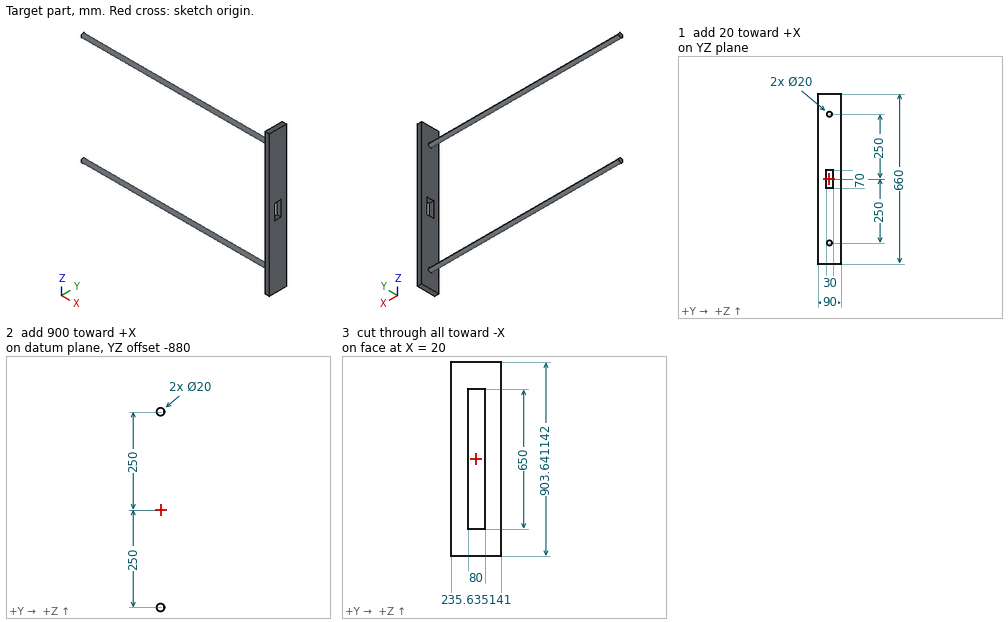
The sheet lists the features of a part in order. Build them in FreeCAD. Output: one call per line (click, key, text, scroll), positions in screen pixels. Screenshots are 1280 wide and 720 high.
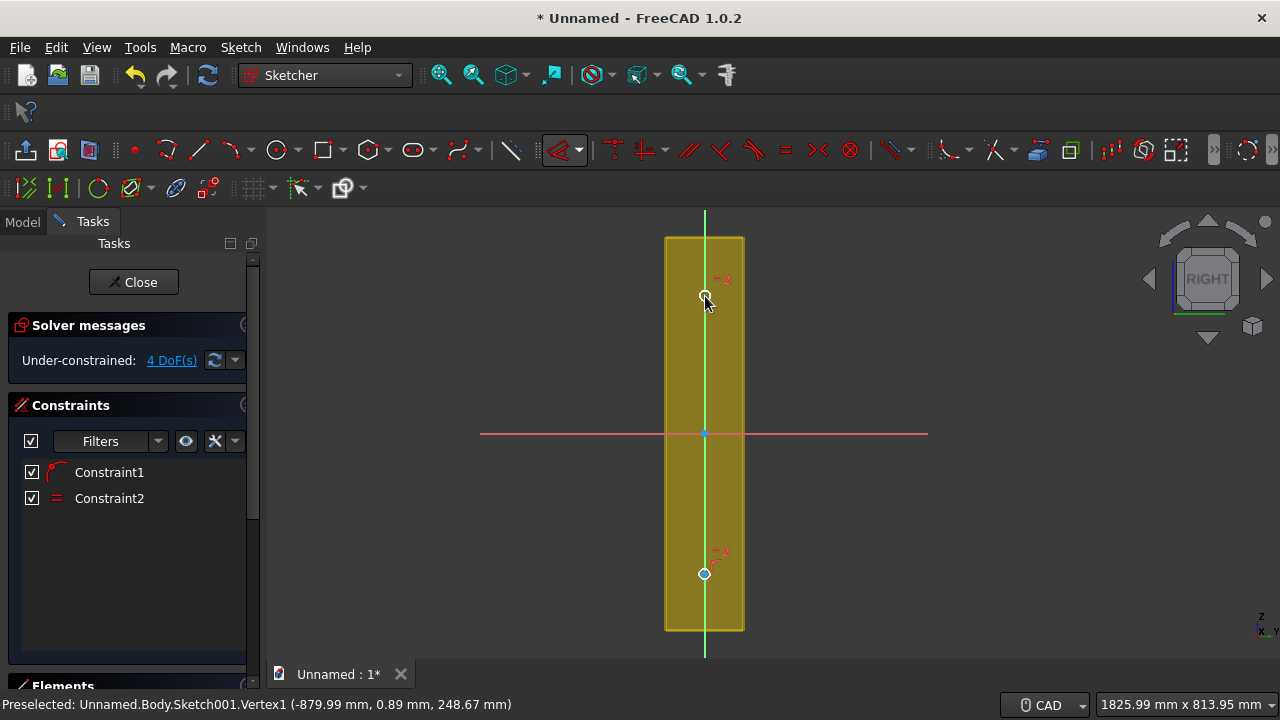
click(705, 518)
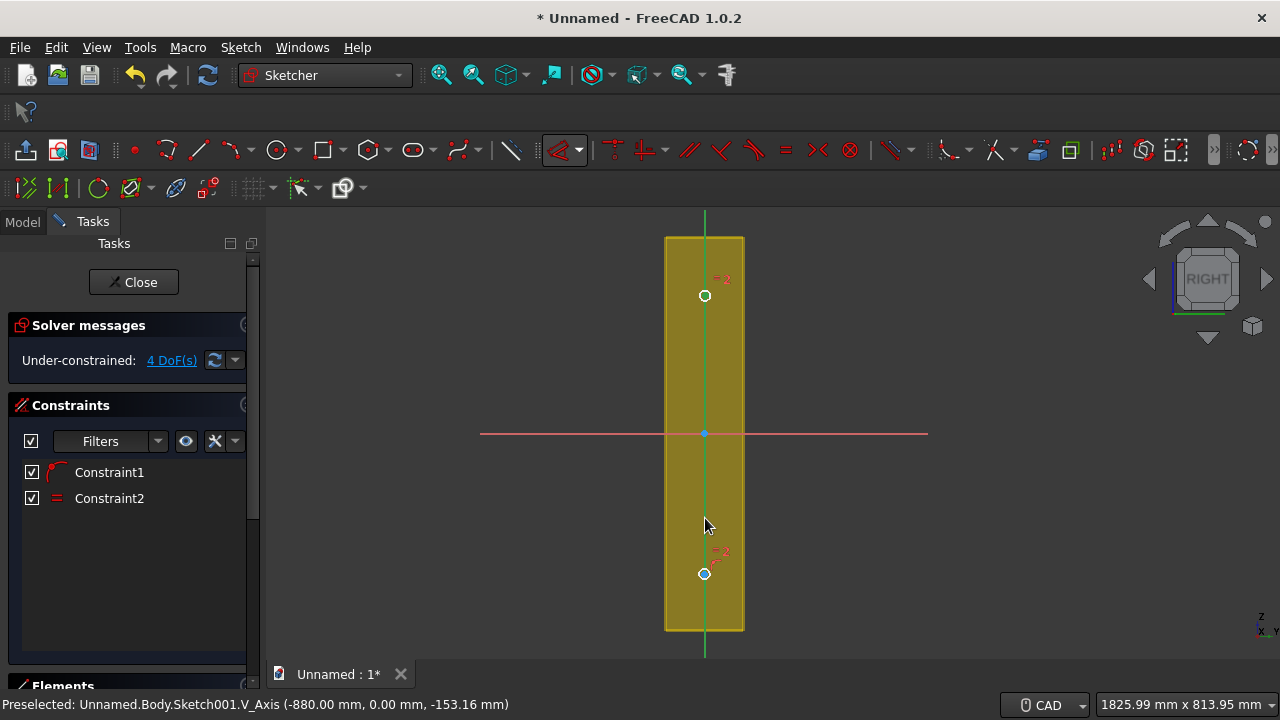
key(c)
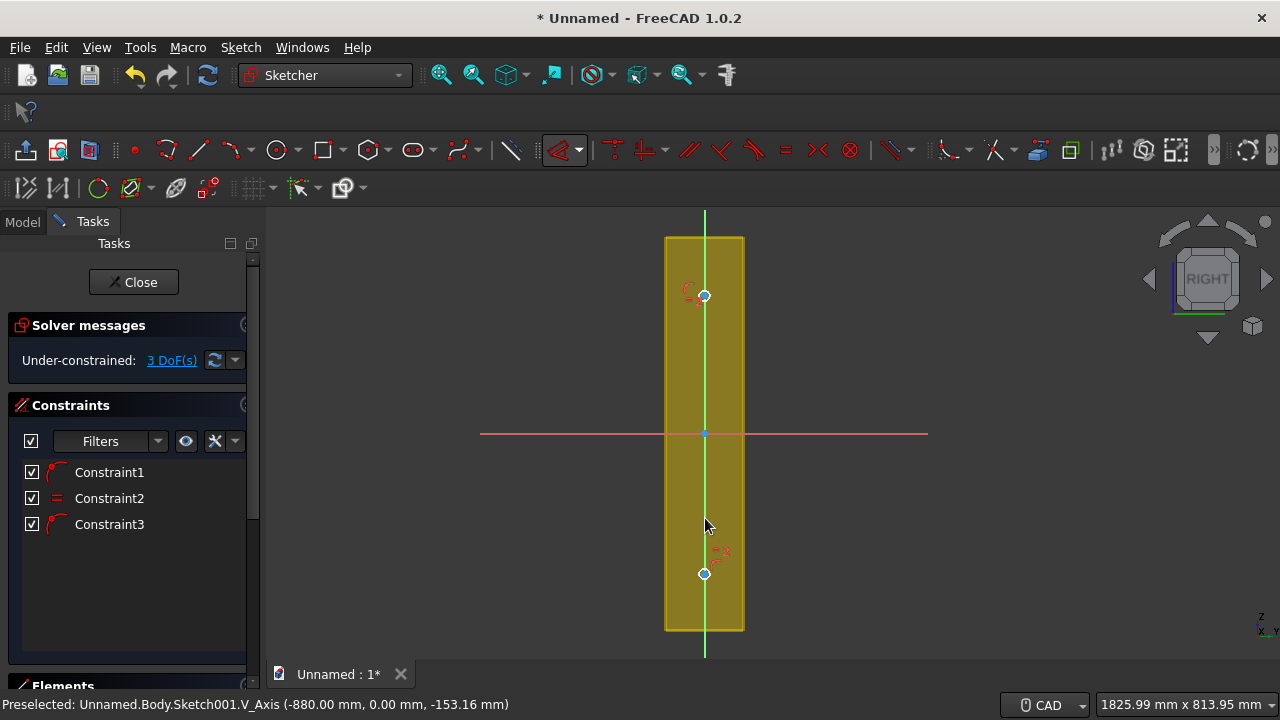
key(d)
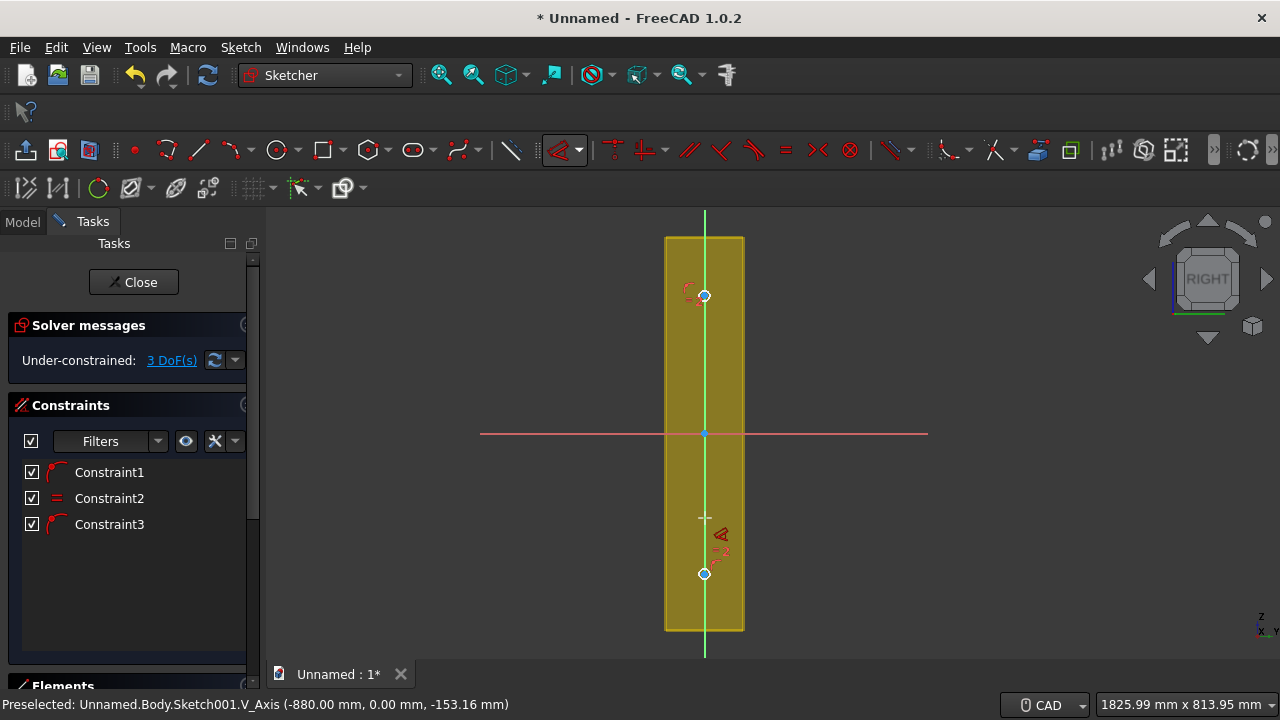
scroll(705, 291, up, 7)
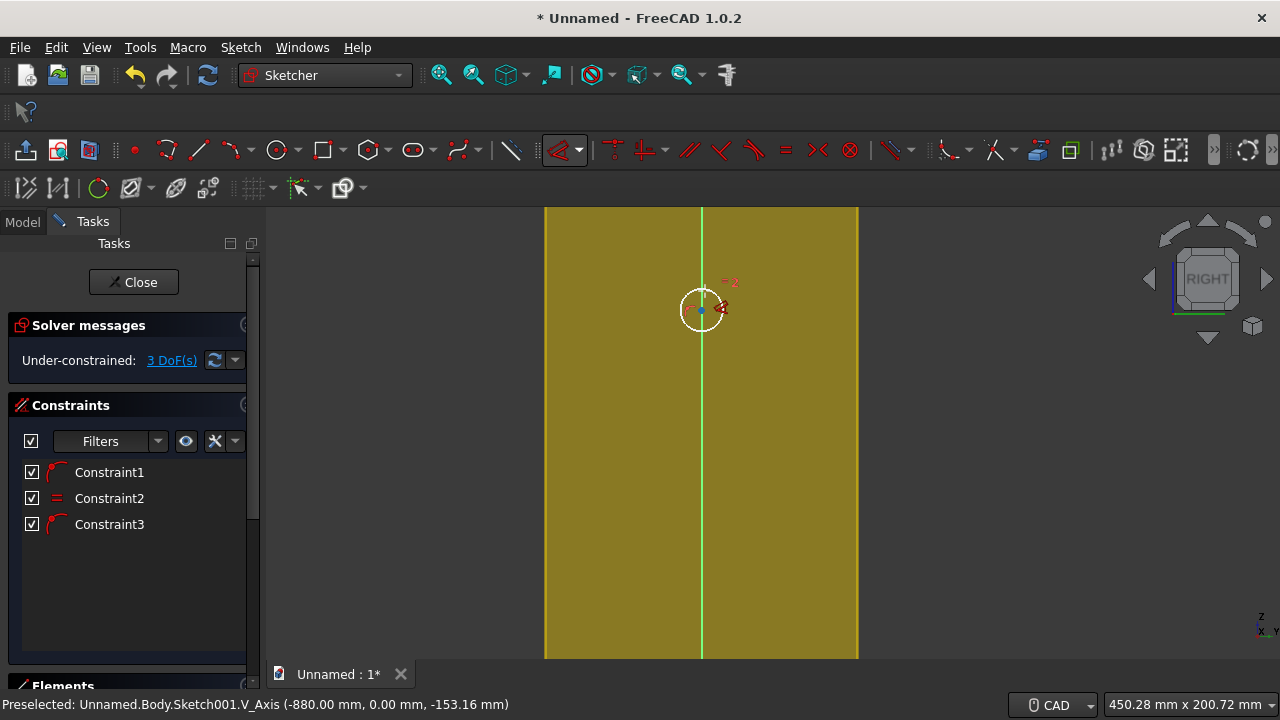
click(702, 289)
click(728, 264)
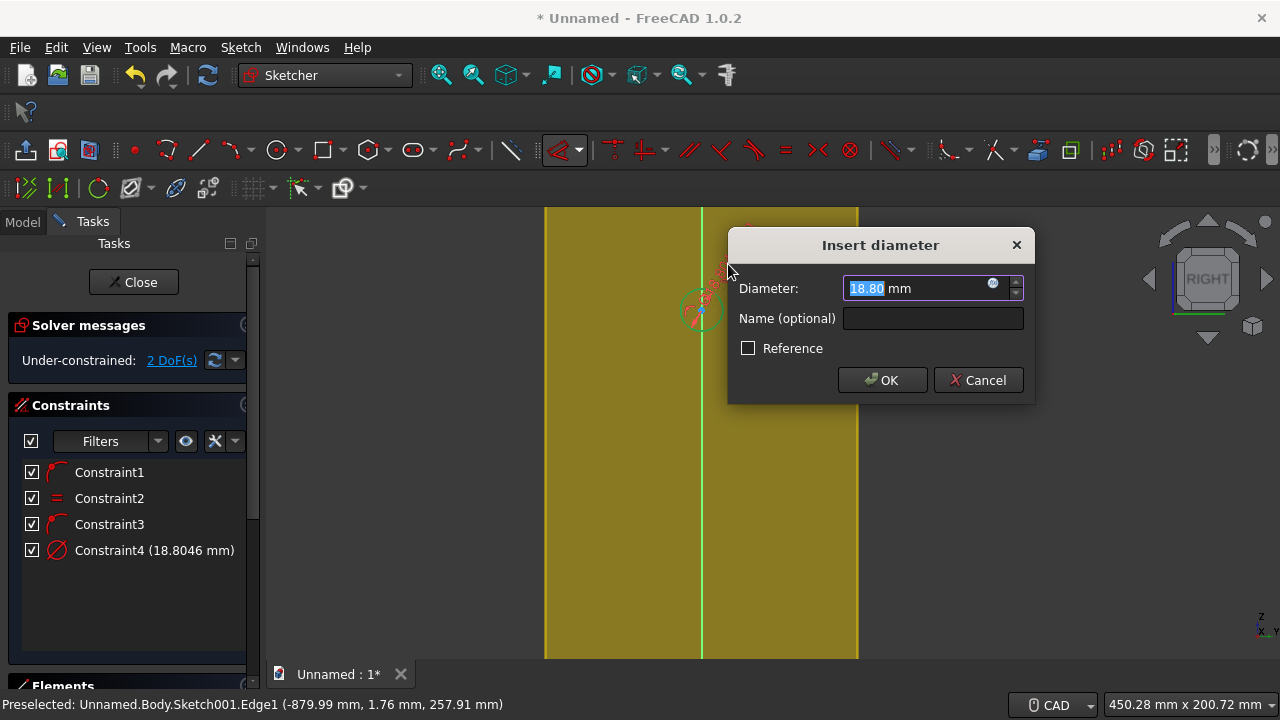
text(20)
key(Return)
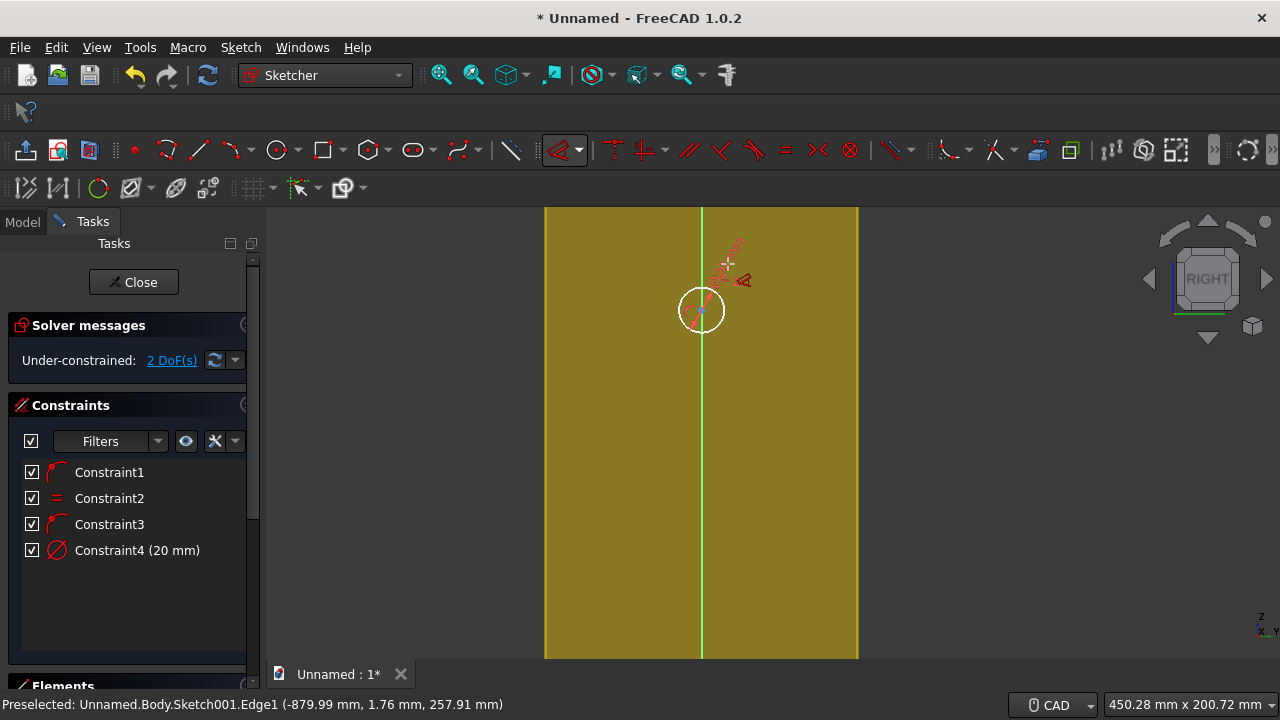
scroll(705, 290, down, 7)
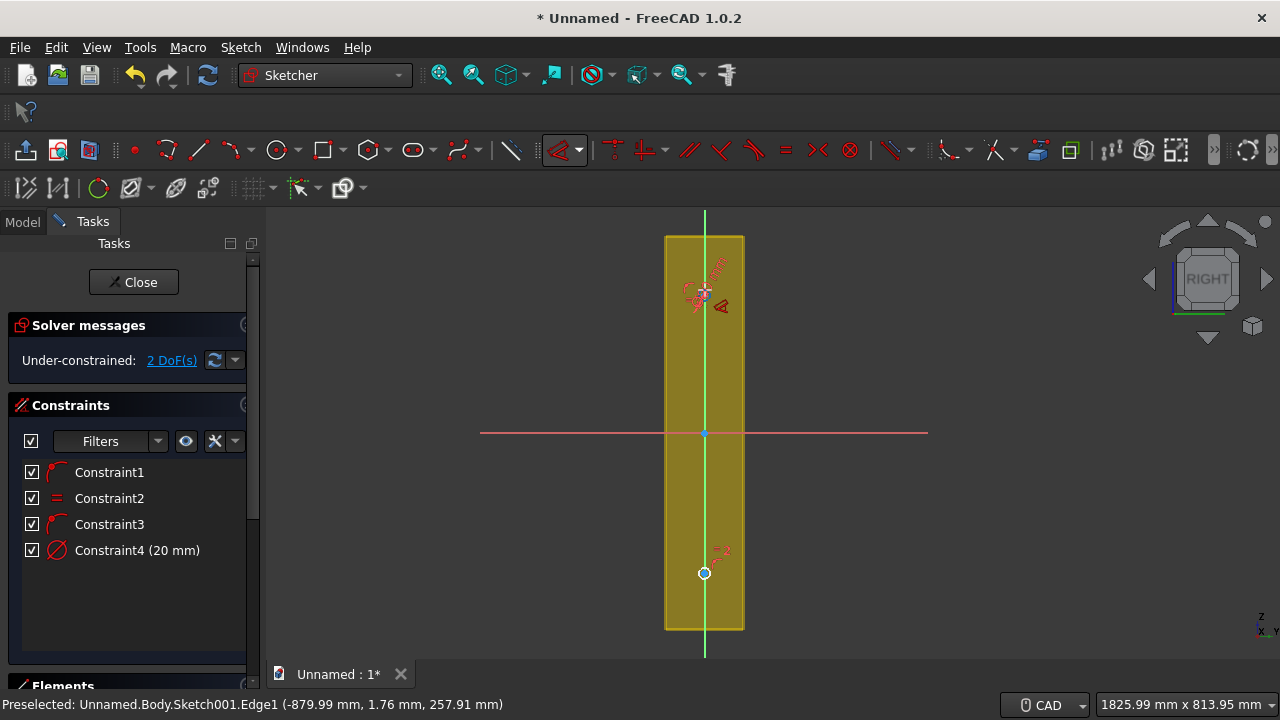
click(705, 295)
click(739, 364)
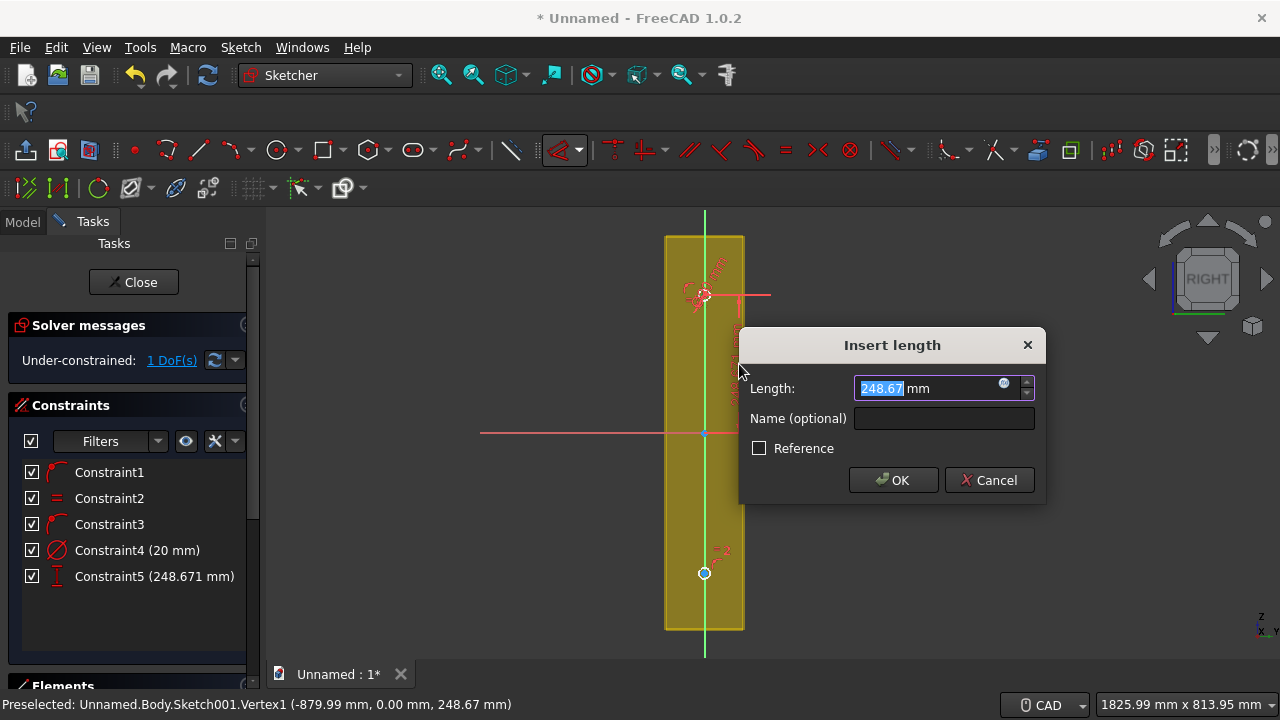
text(250)
key(Return)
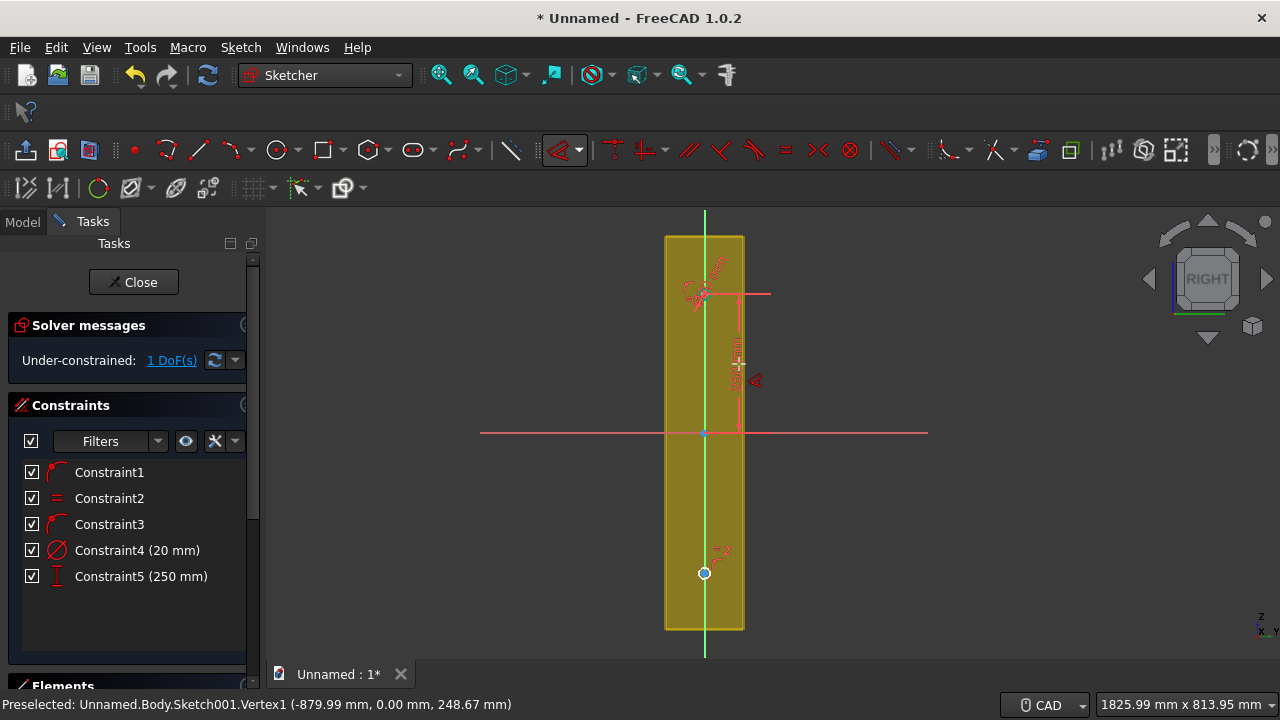
click(705, 573)
click(739, 503)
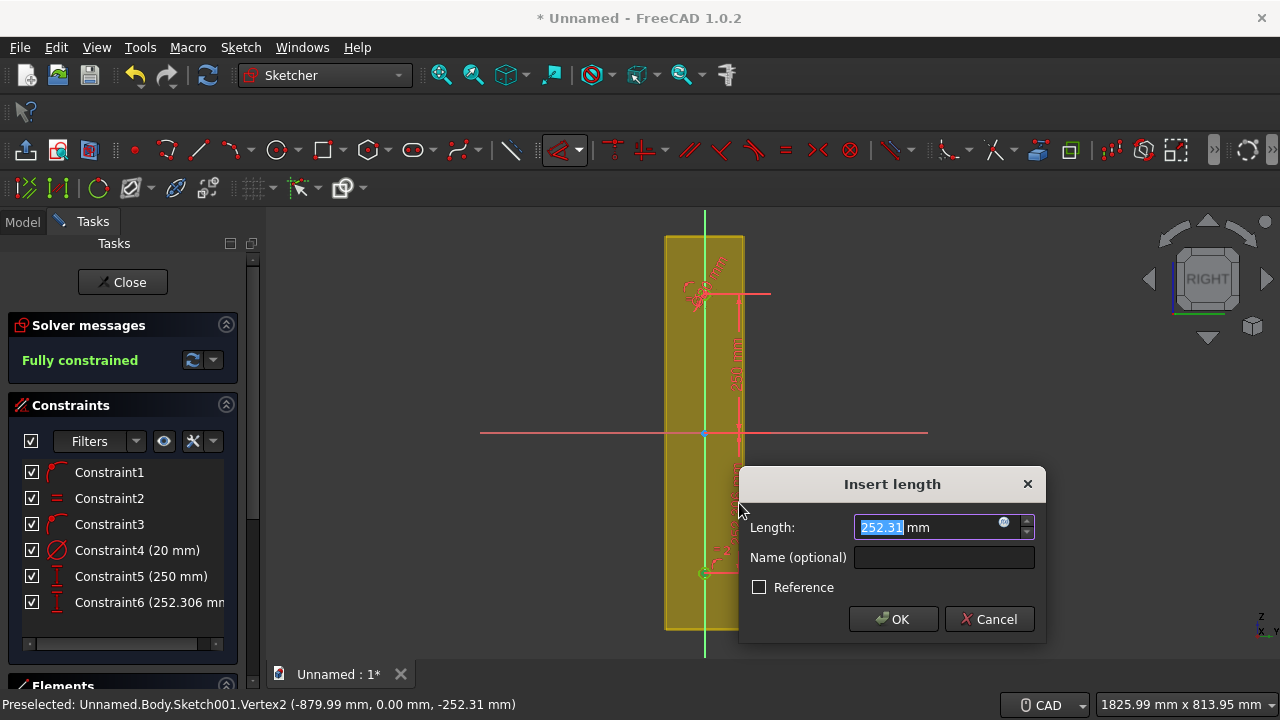
text(250)
key(Return)
key(Escape)